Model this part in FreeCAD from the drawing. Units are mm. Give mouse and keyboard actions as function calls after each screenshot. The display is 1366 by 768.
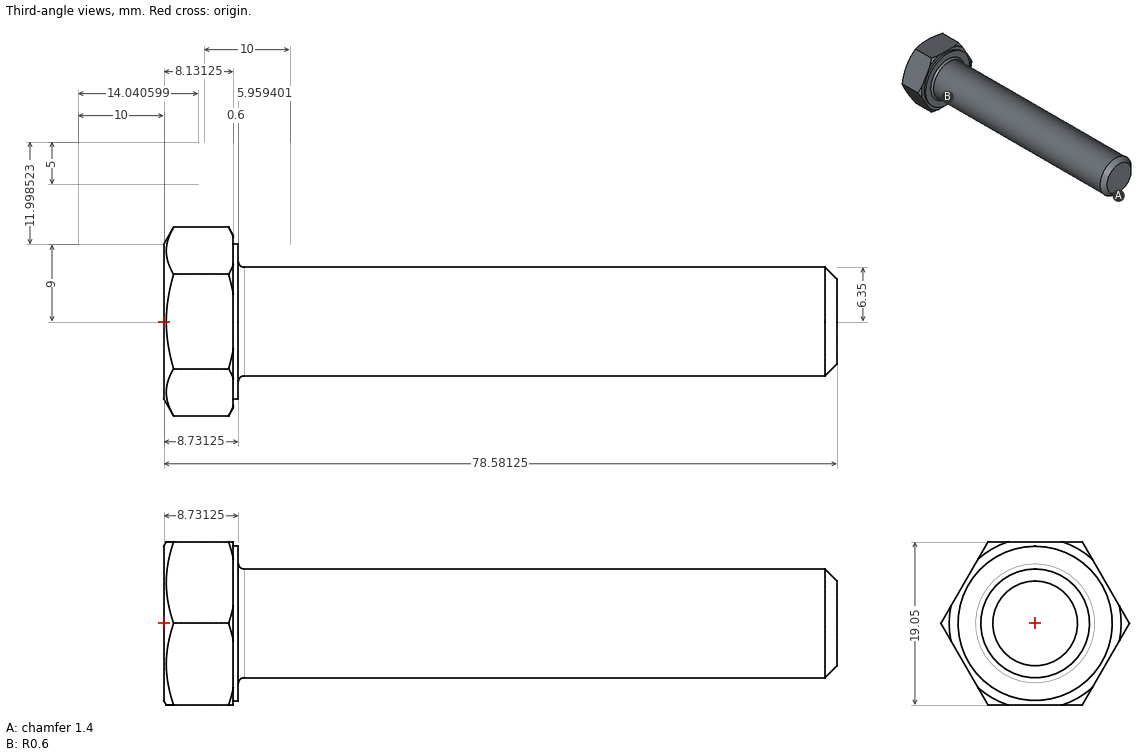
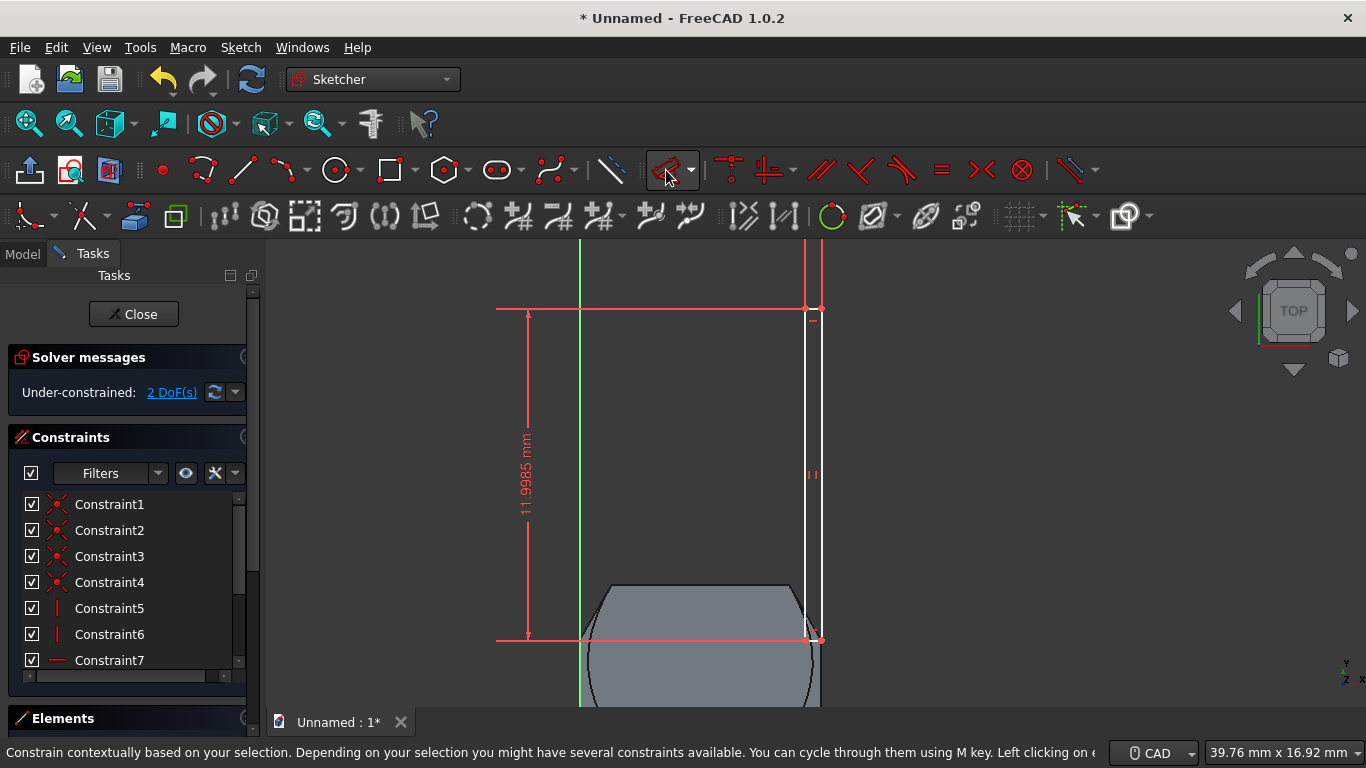
click(805, 641)
click(546, 660)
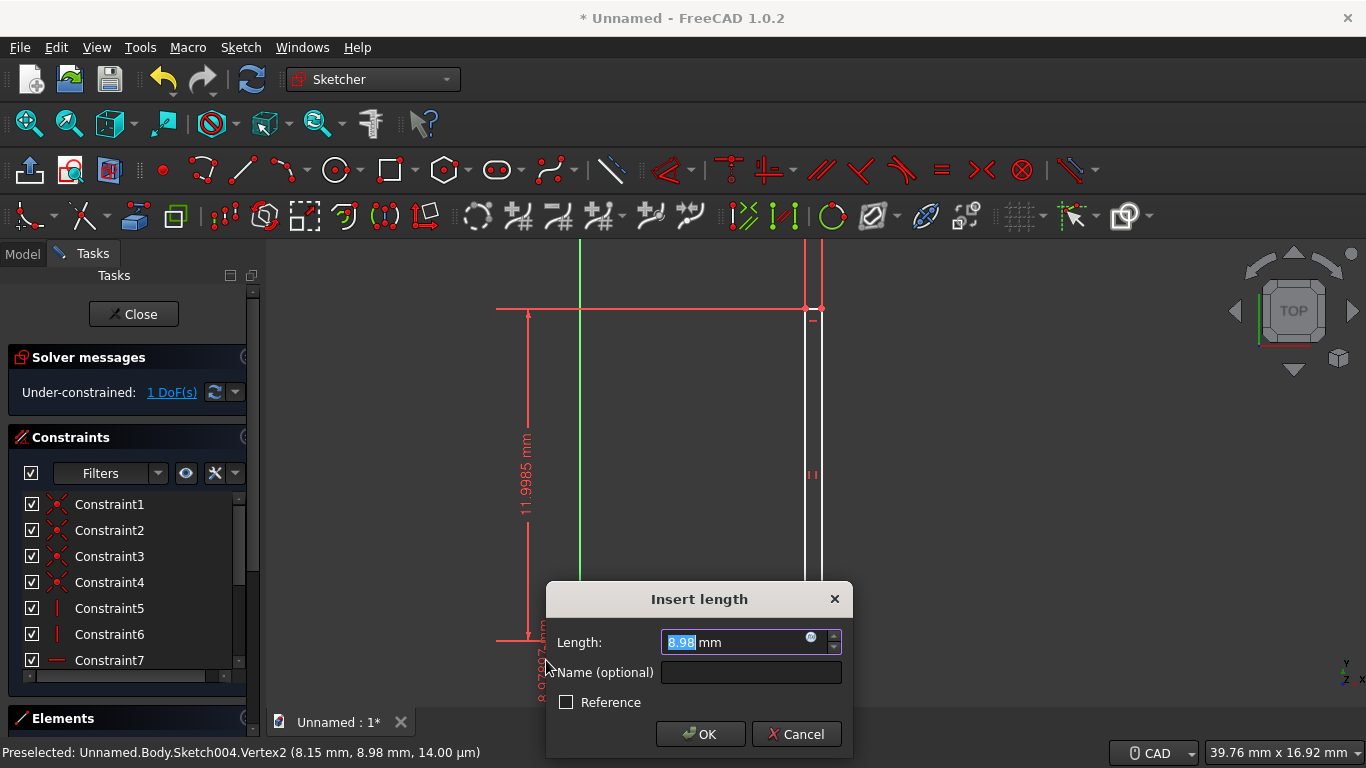
text(9)
key(Return)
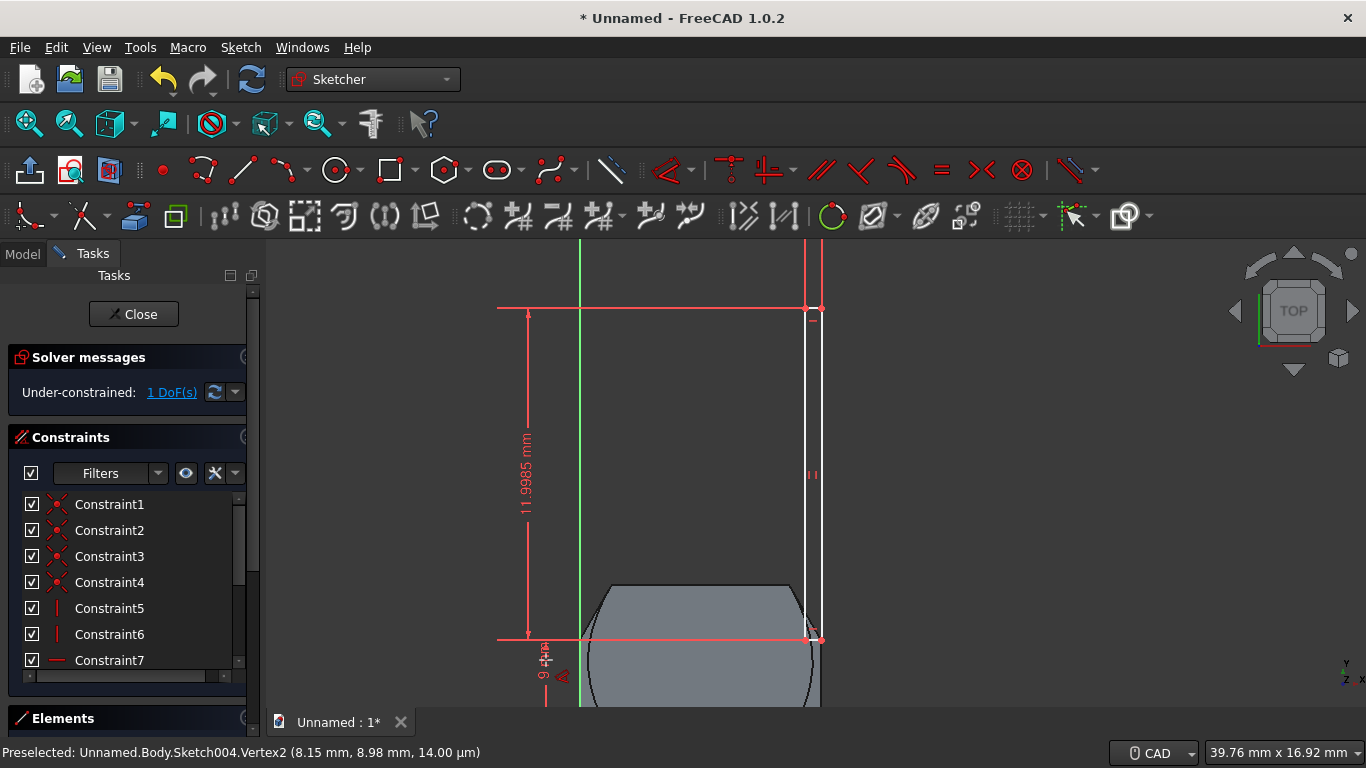
click(805, 308)
click(692, 274)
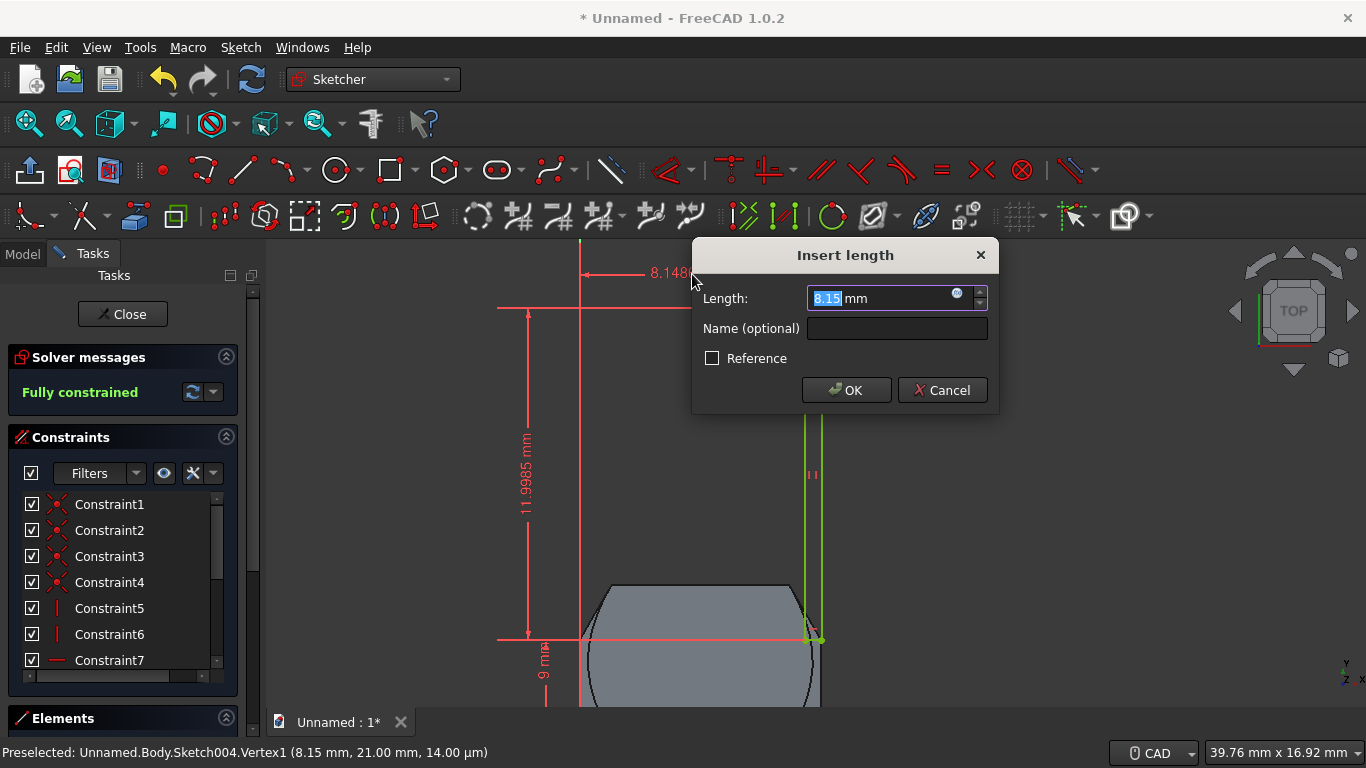
text(8.13125)
key(Return)
key(Escape)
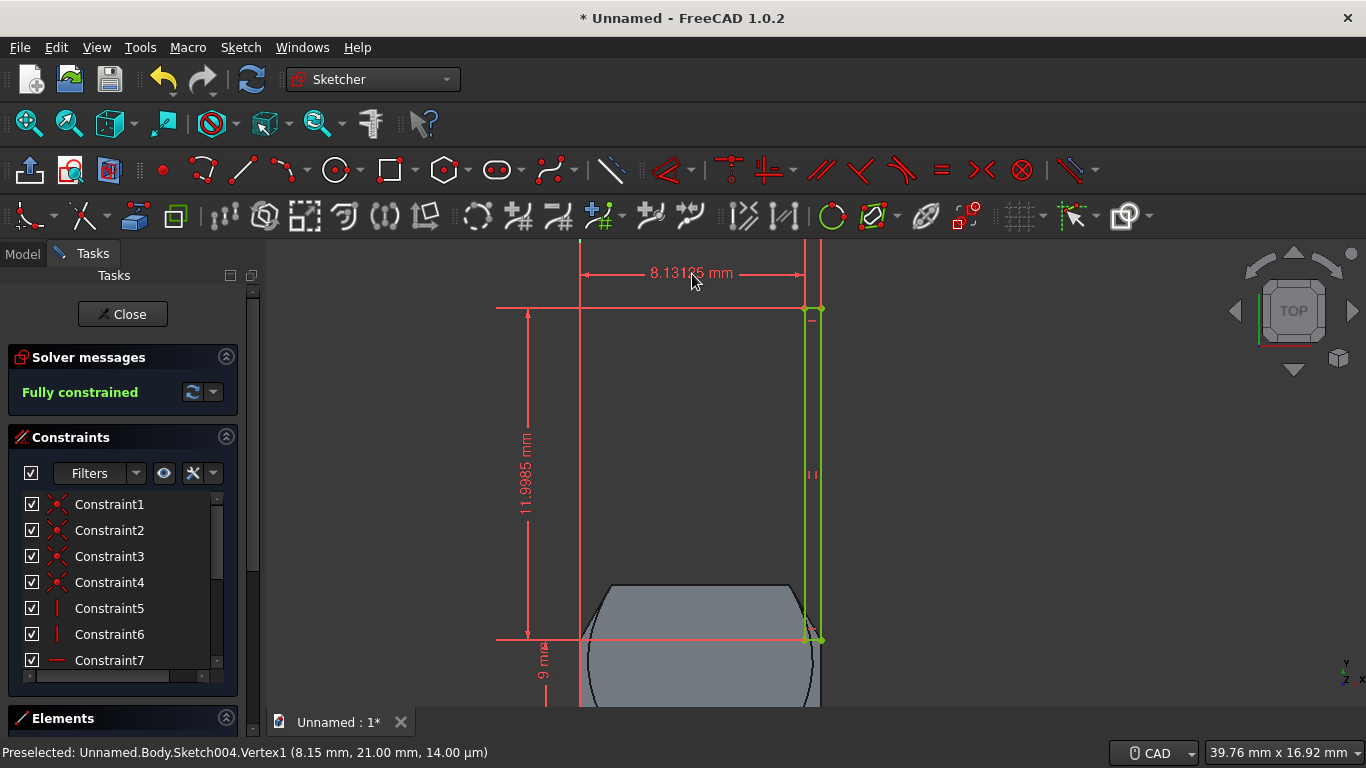
click(123, 314)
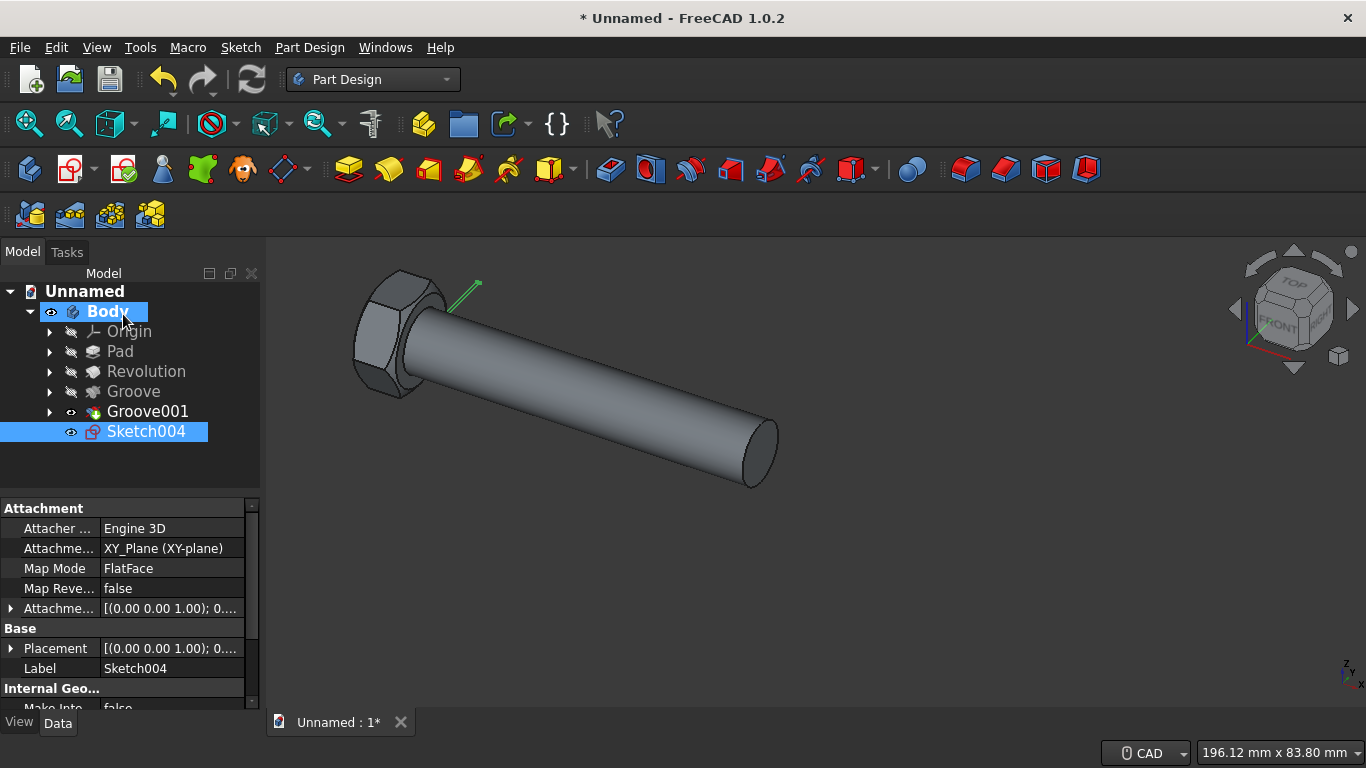
click(692, 170)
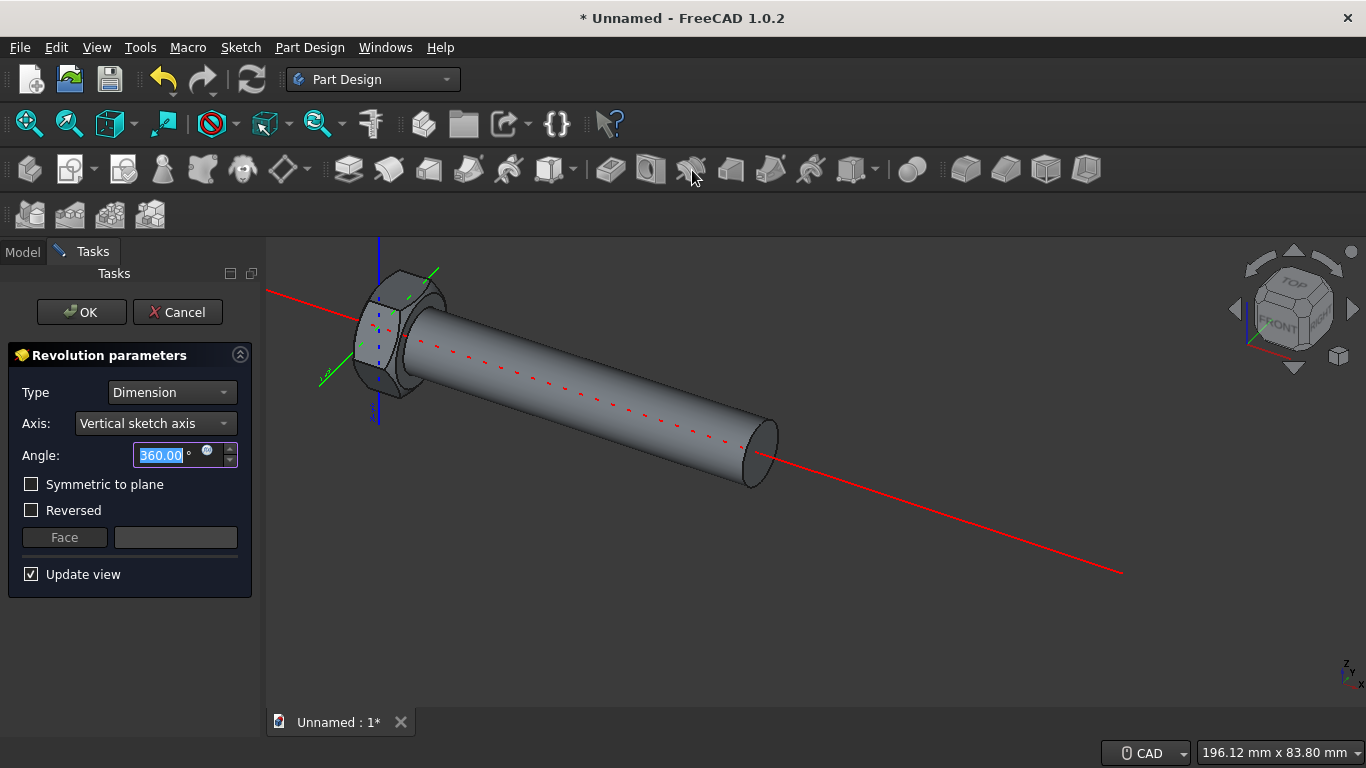
click(156, 424)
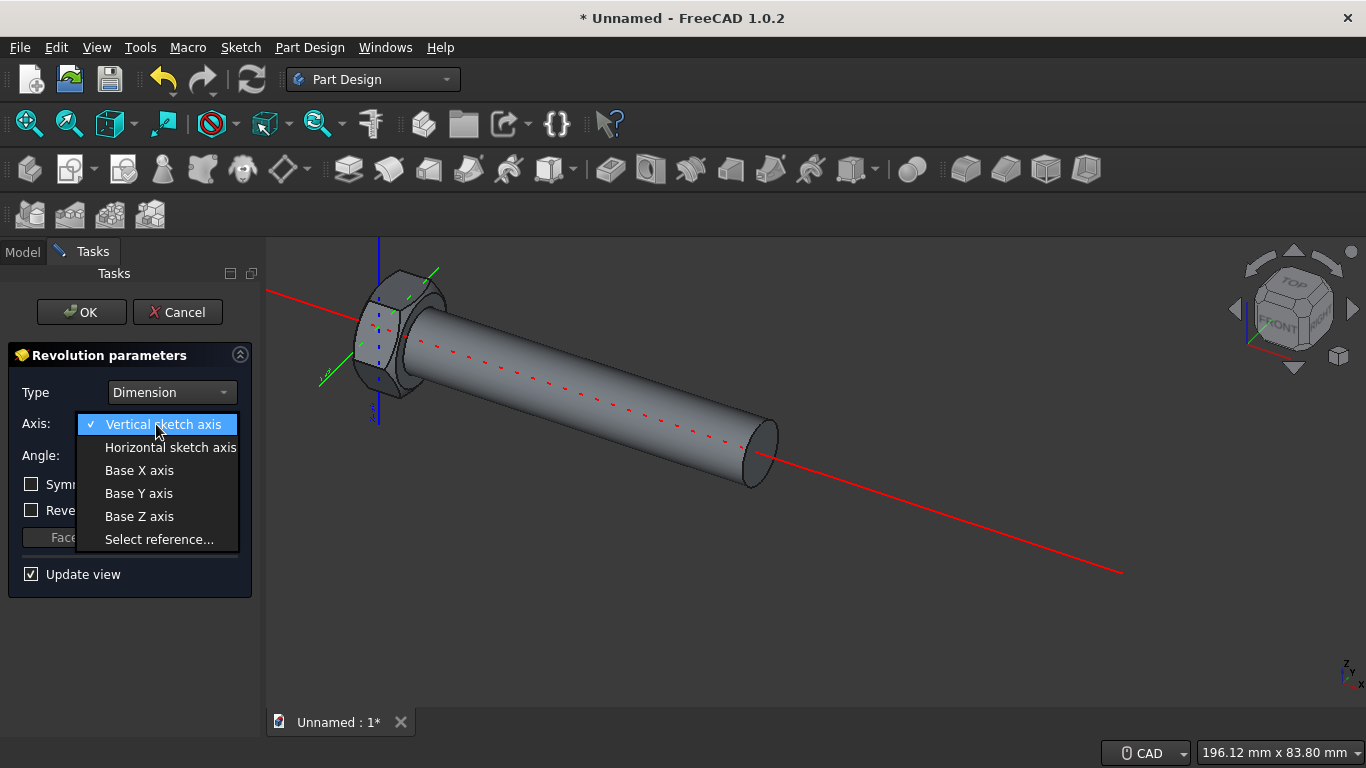
click(156, 448)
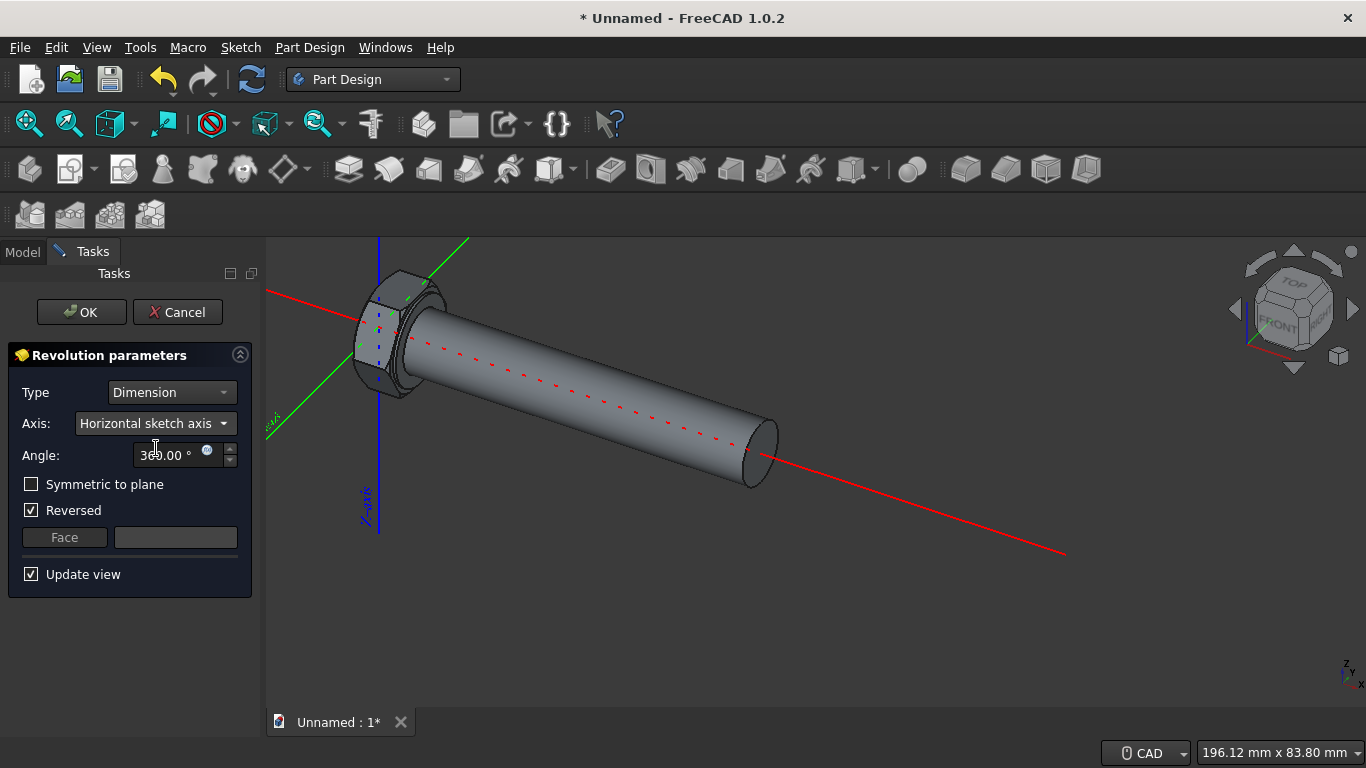
click(82, 312)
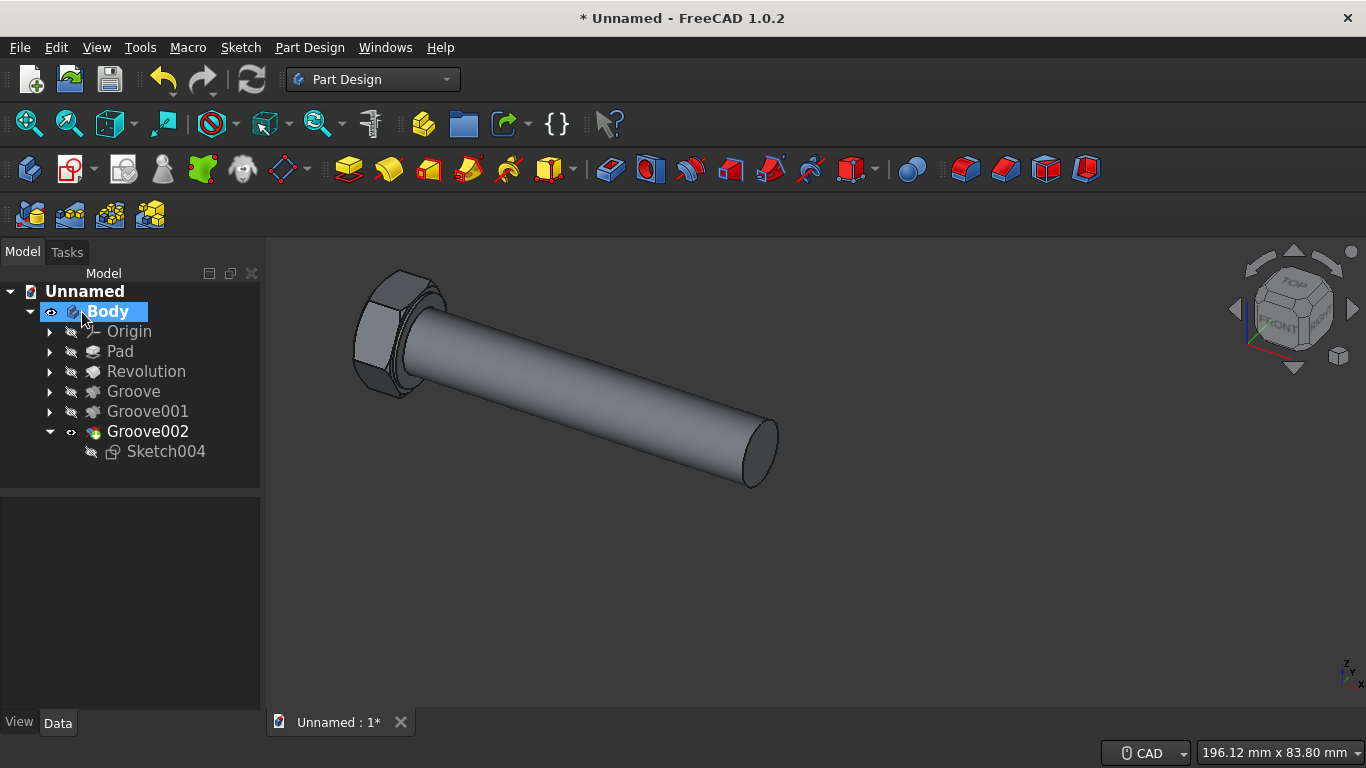
click(743, 470)